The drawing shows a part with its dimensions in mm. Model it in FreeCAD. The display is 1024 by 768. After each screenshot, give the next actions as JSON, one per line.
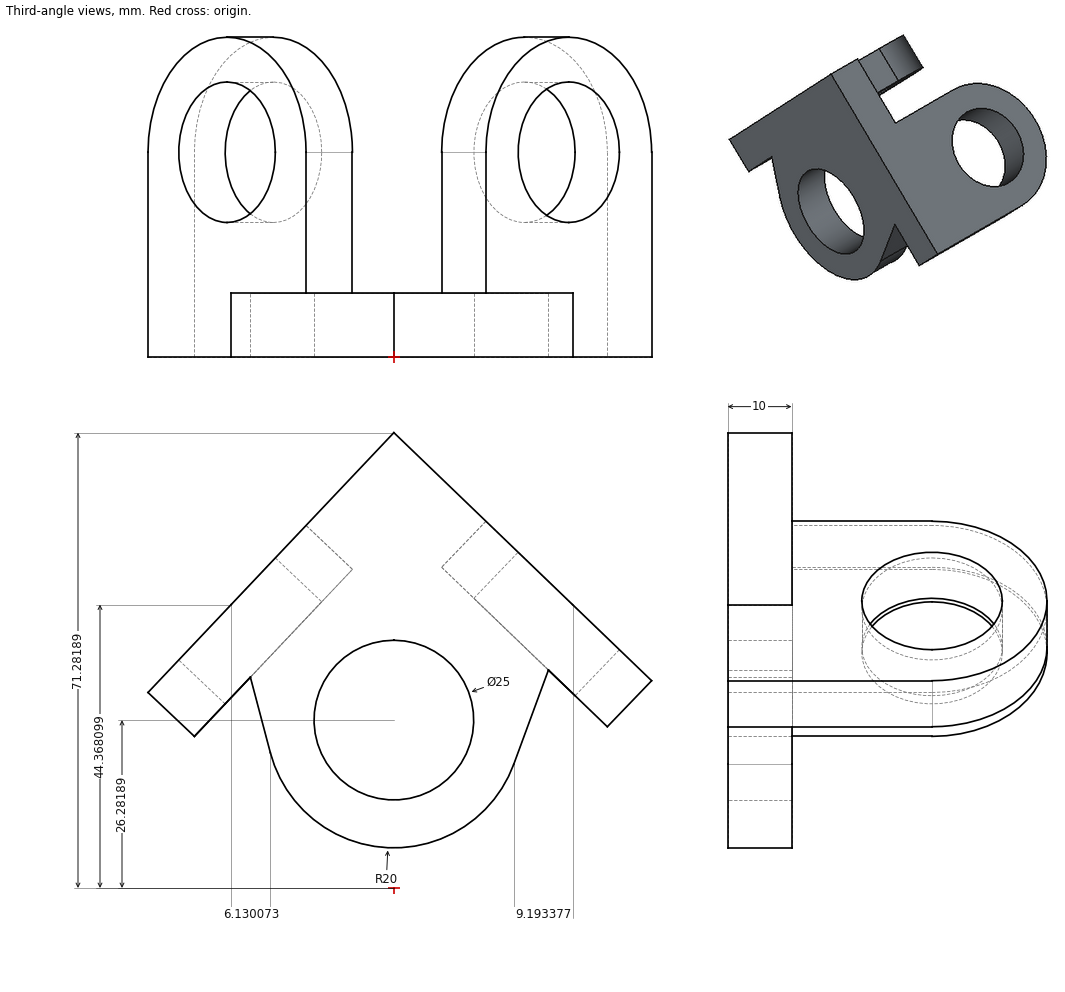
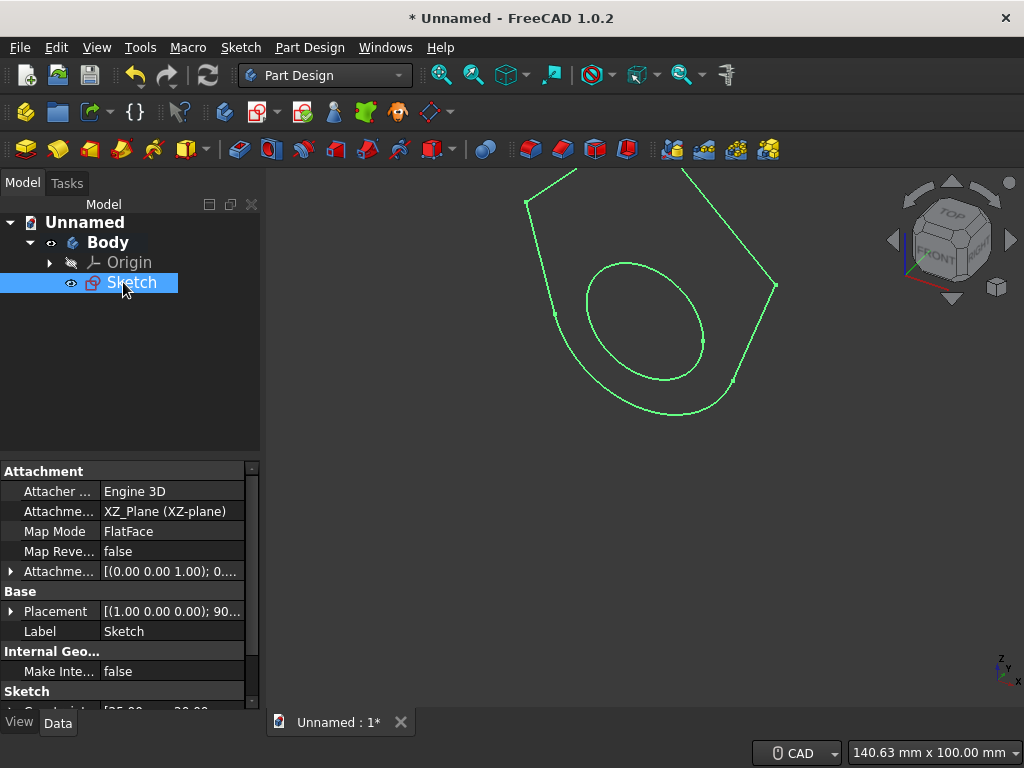
{"action": "left_click", "coordinate": [26, 150]}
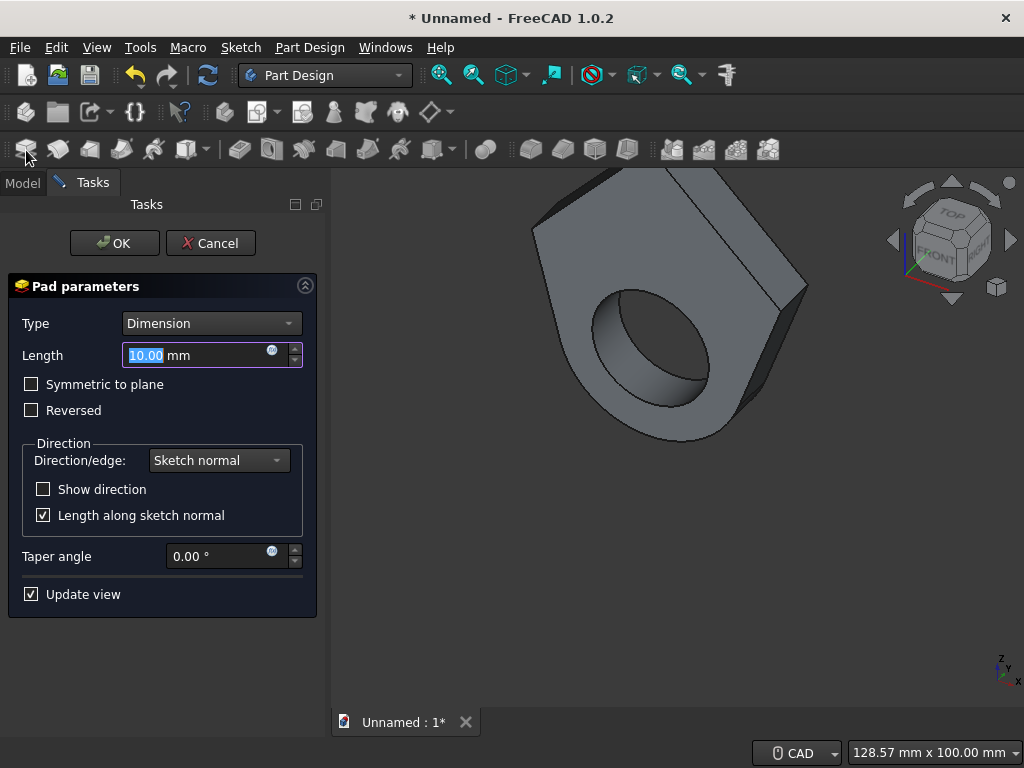
{"action": "type", "text": "10"}
{"action": "key", "text": "Tab"}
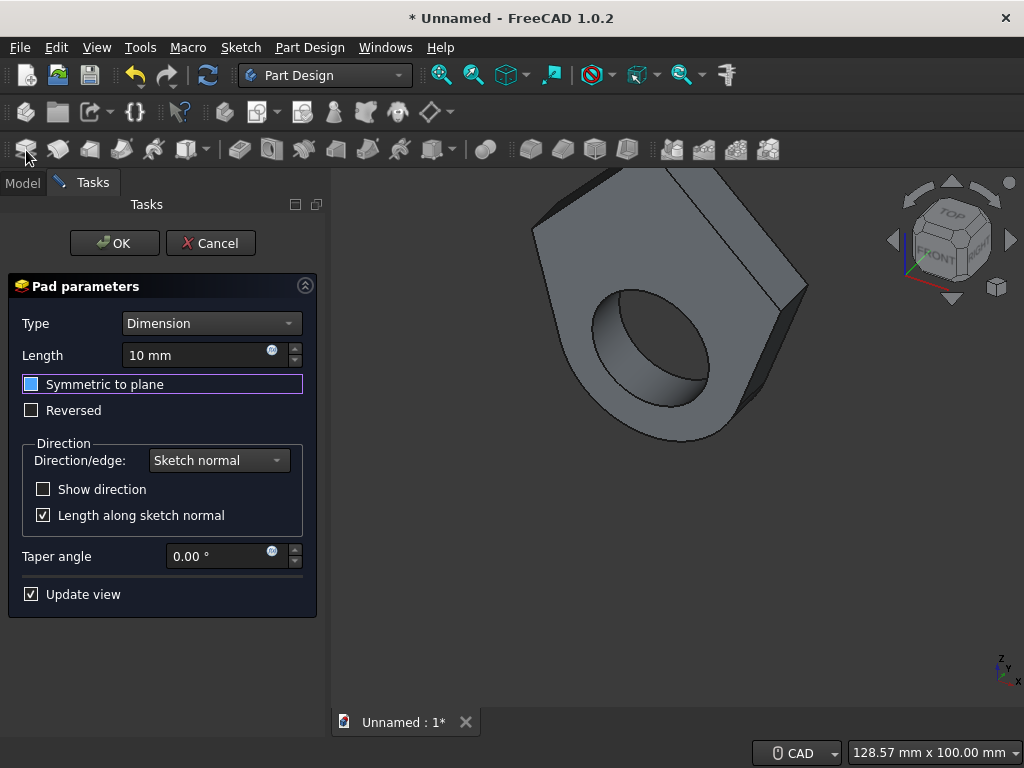
{"action": "left_click", "coordinate": [30, 410]}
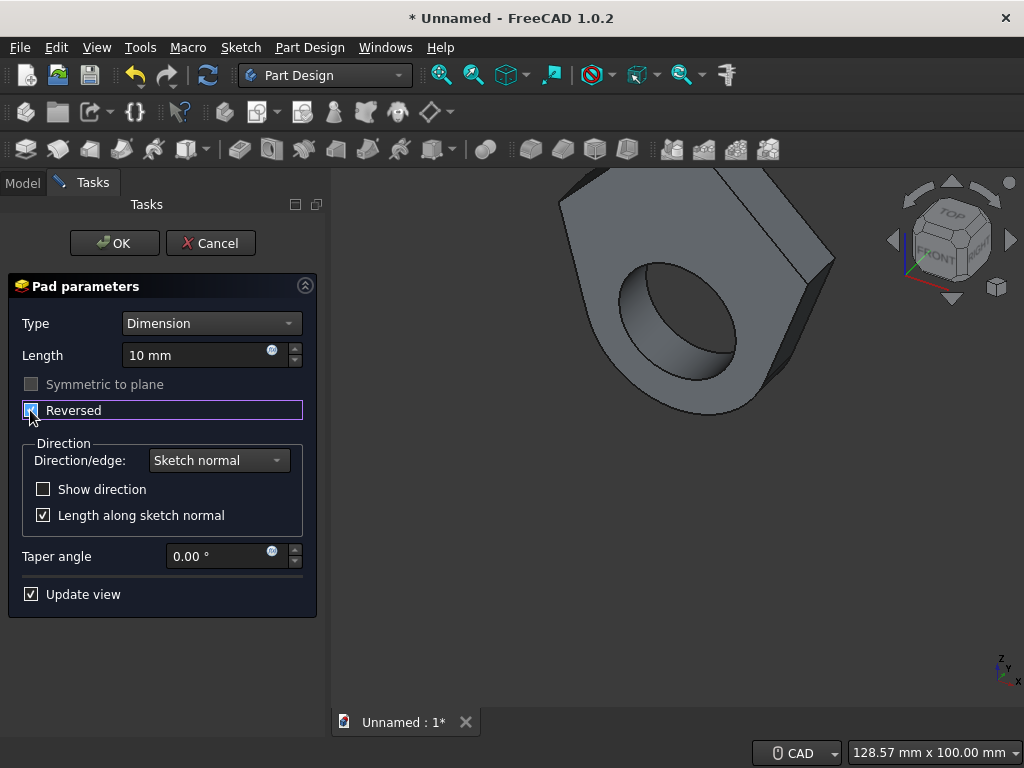
{"action": "left_click", "coordinate": [115, 243]}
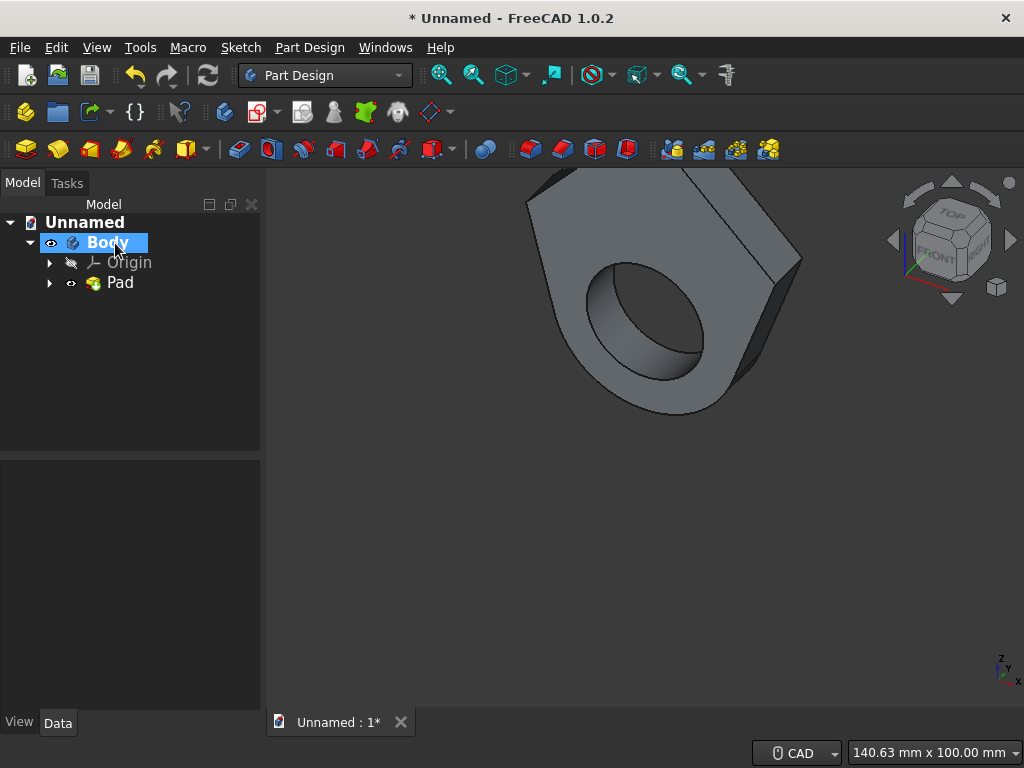
{"action": "left_click", "coordinate": [442, 76]}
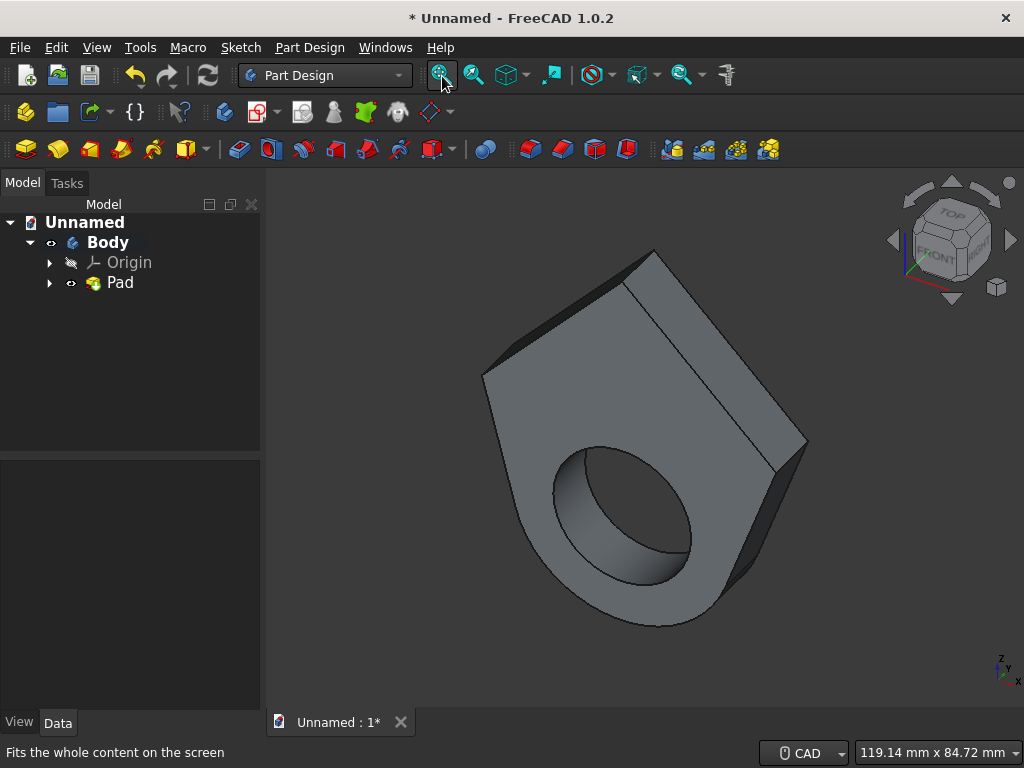
{"action": "left_click", "coordinate": [737, 388]}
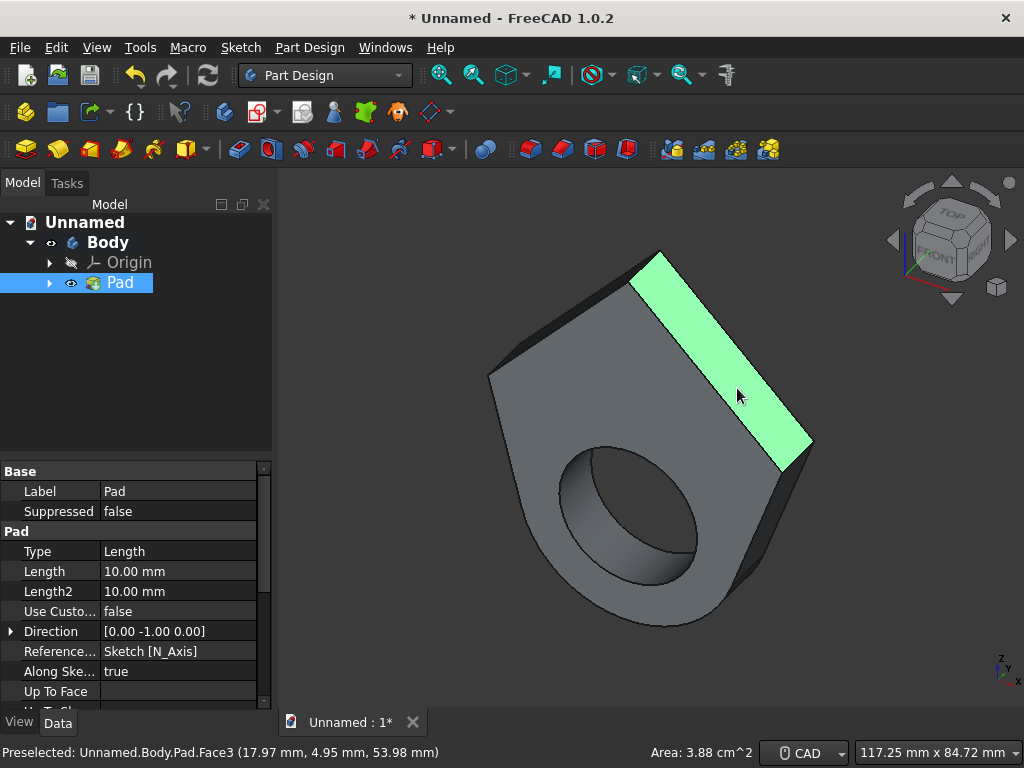
{"action": "left_click", "coordinate": [258, 112]}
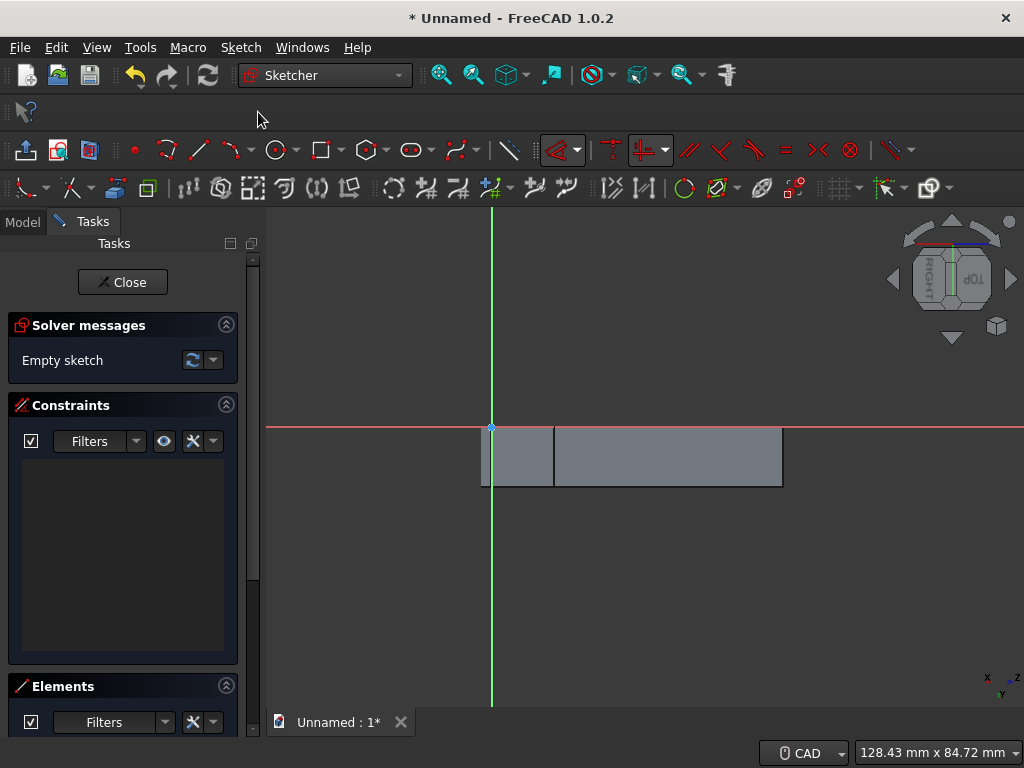
{"action": "scroll", "coordinate": [656, 235], "scroll_direction": "down", "scroll_amount": 1}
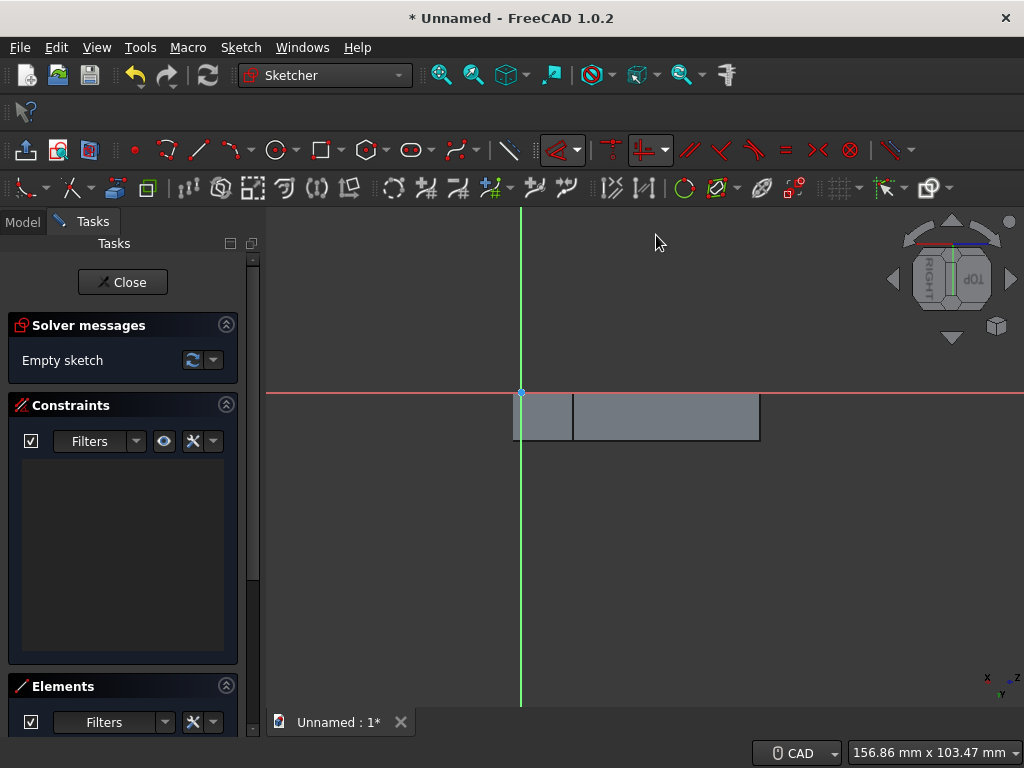
{"action": "left_click", "coordinate": [168, 150]}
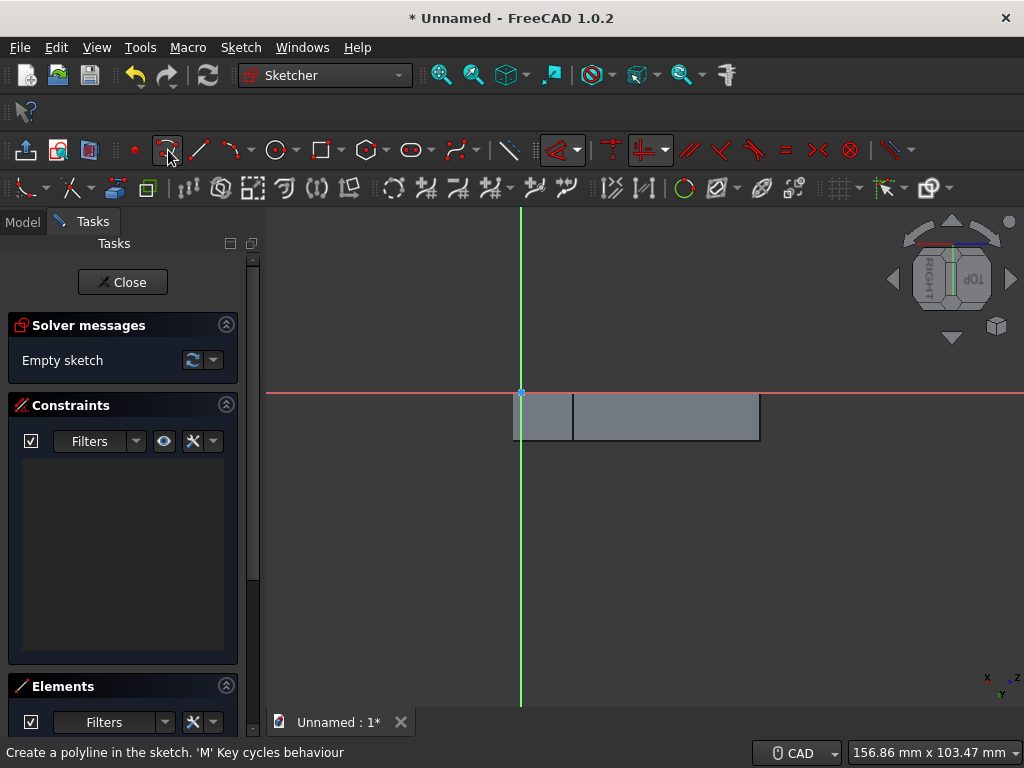
{"action": "left_click", "coordinate": [664, 547]}
{"action": "left_click", "coordinate": [664, 393]}
{"action": "left_click", "coordinate": [490, 402]}
{"action": "left_click", "coordinate": [490, 547]}
{"action": "right_click", "coordinate": [490, 547]}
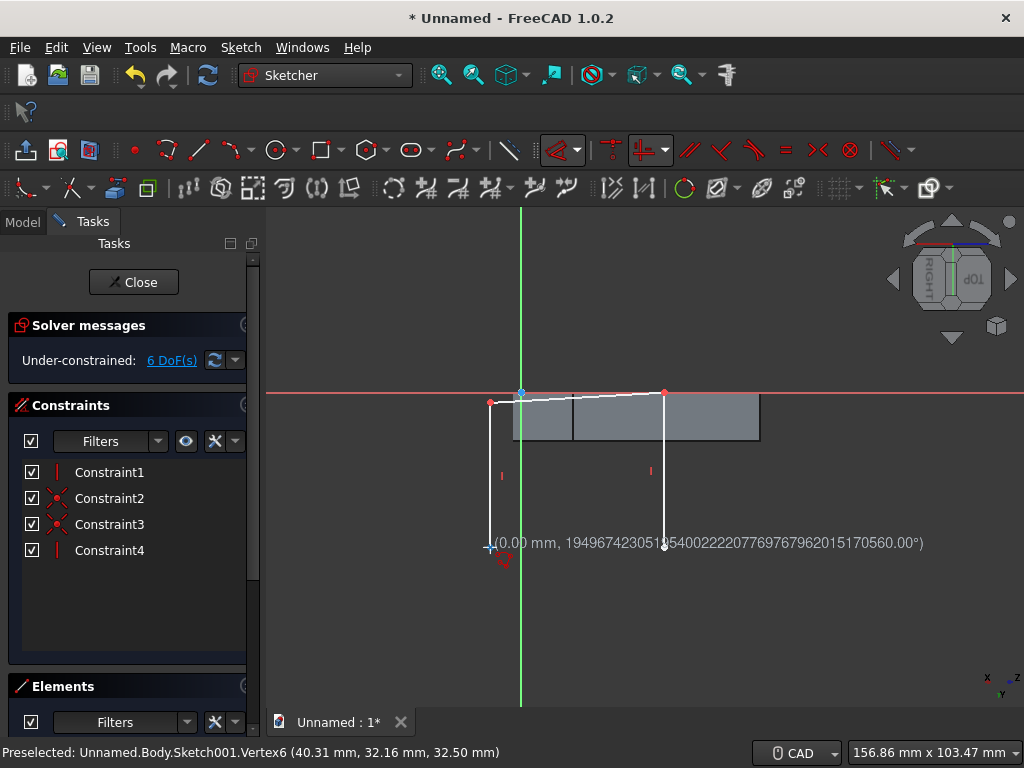
{"action": "left_click", "coordinate": [232, 150]}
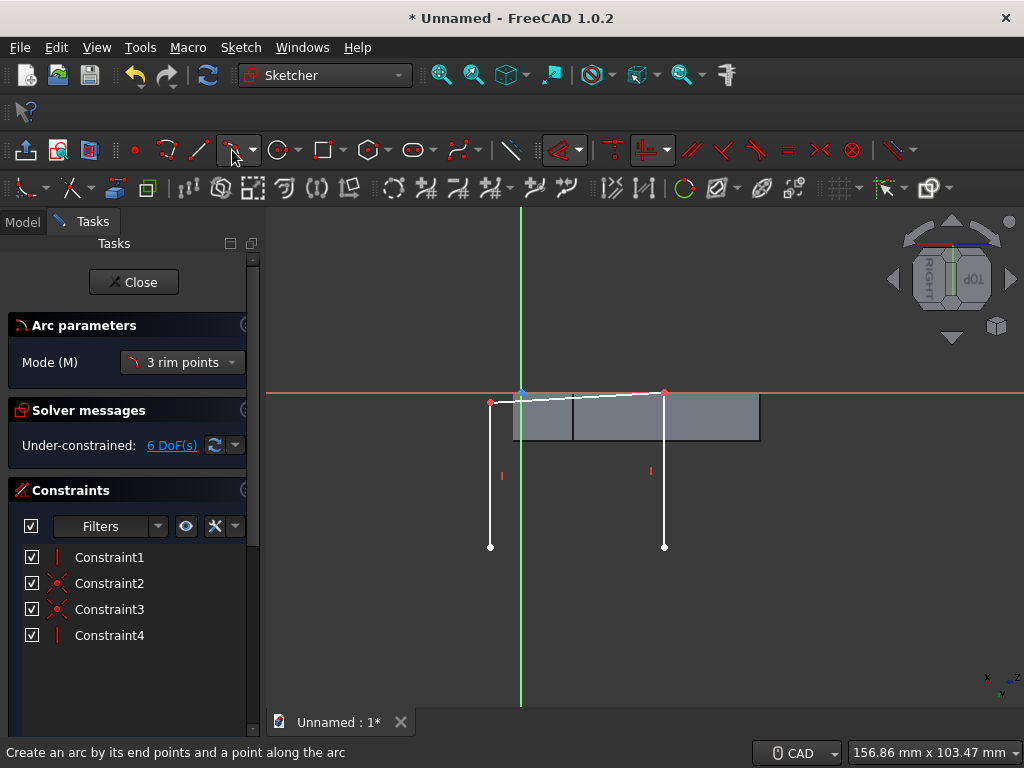
{"action": "left_click", "coordinate": [490, 548]}
{"action": "left_click", "coordinate": [664, 548]}
{"action": "left_click", "coordinate": [577, 634]}